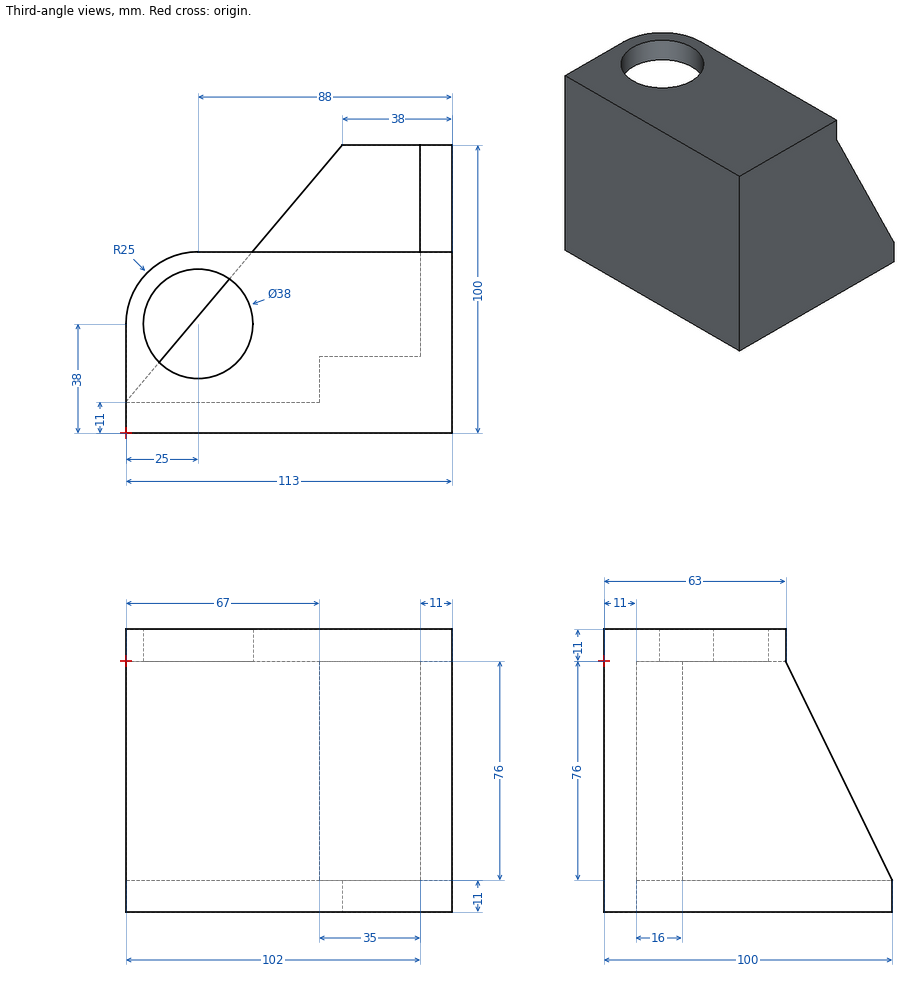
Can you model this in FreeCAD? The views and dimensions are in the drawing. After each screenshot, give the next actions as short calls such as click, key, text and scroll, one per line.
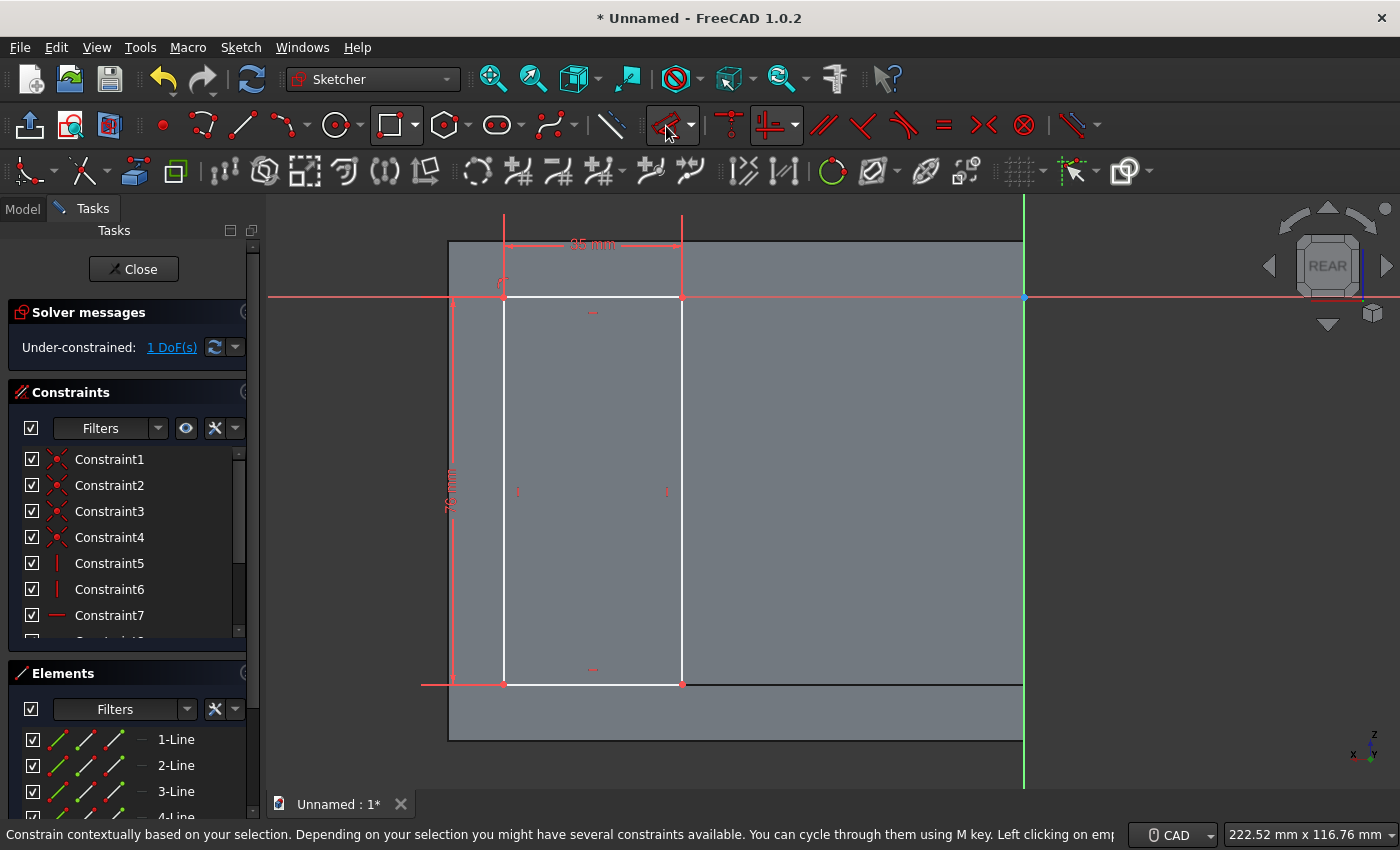
click(682, 685)
click(853, 719)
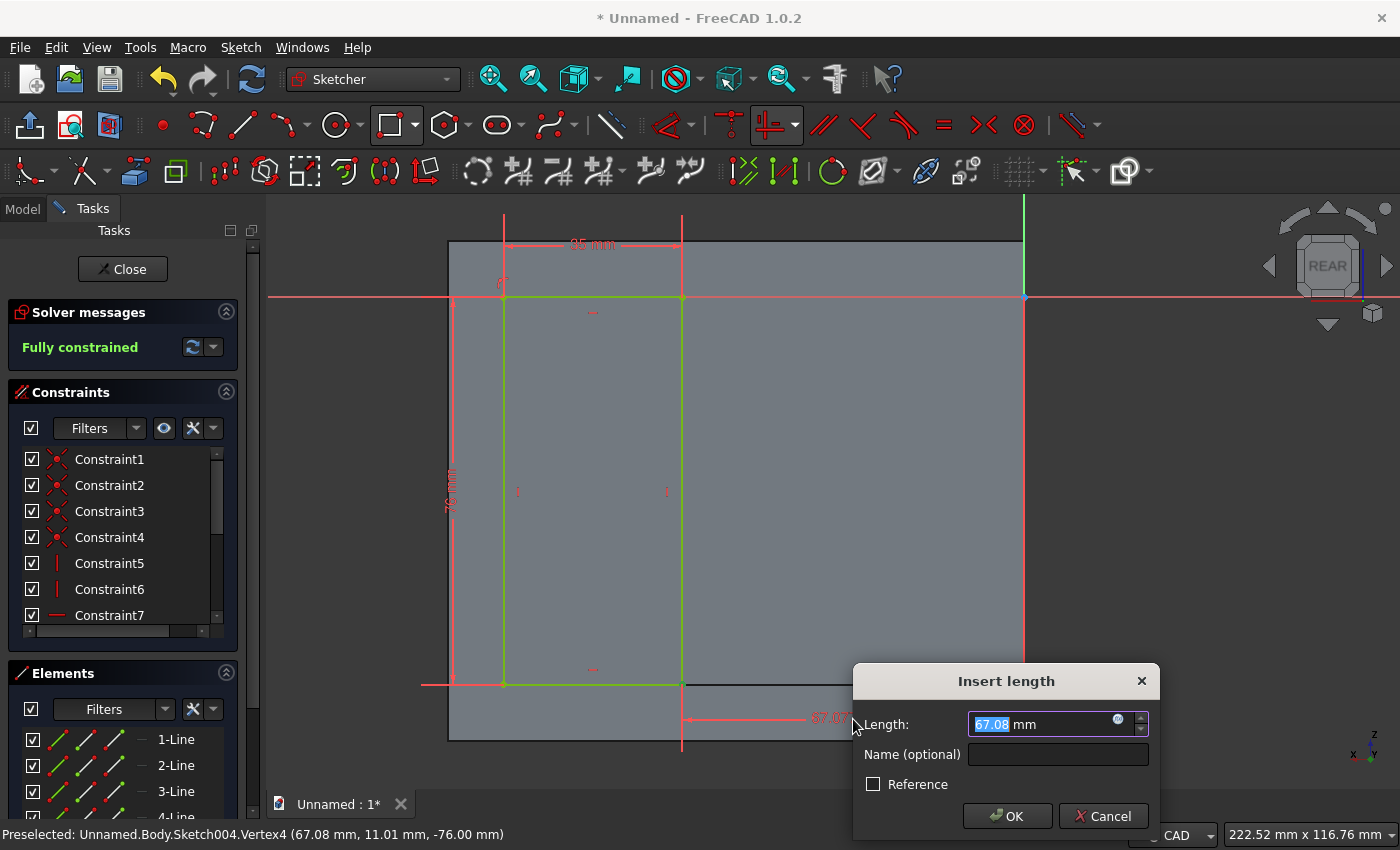
text(67)
key(Return)
key(Escape)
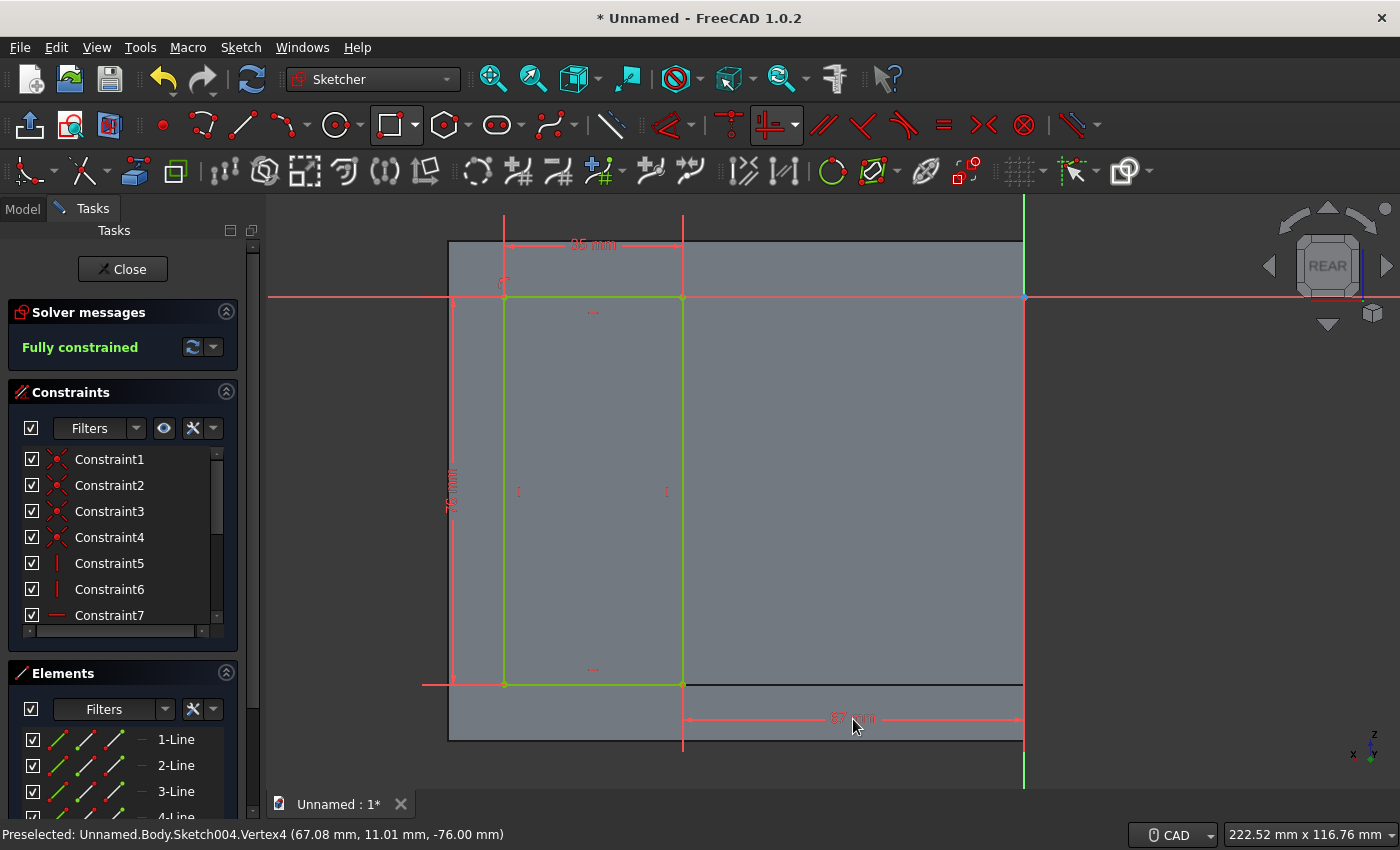
click(123, 269)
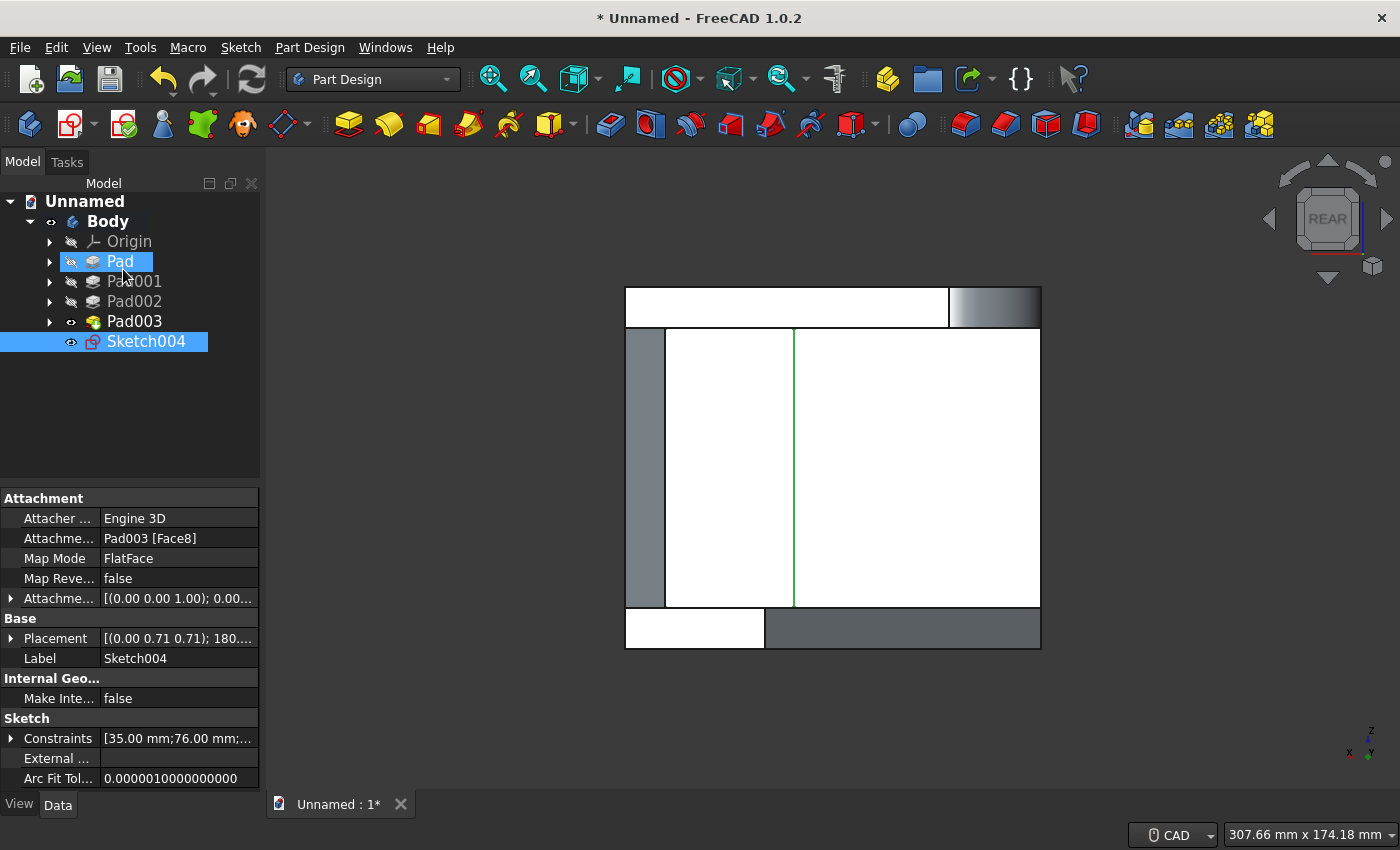
click(350, 124)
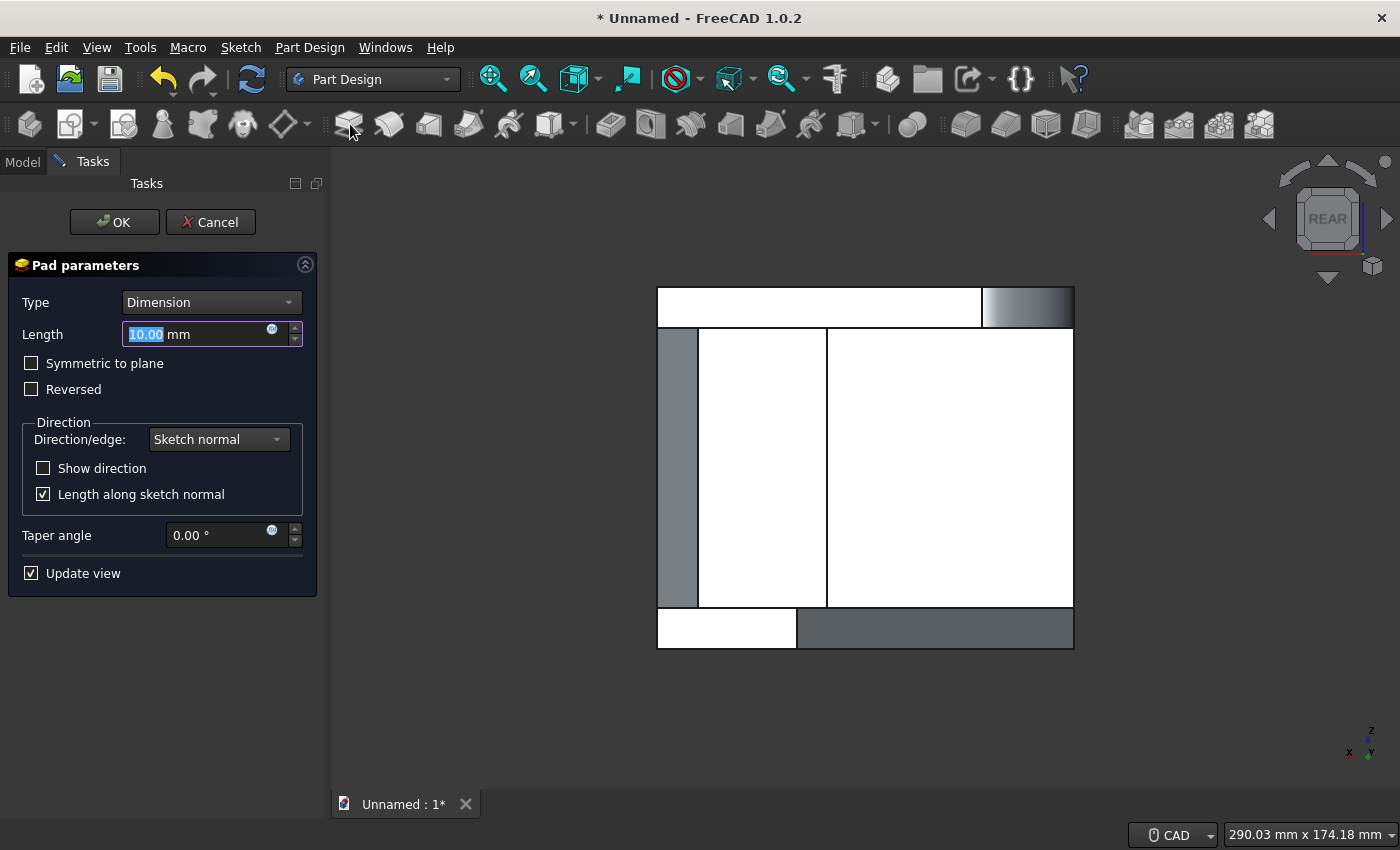
text(16)
key(Tab)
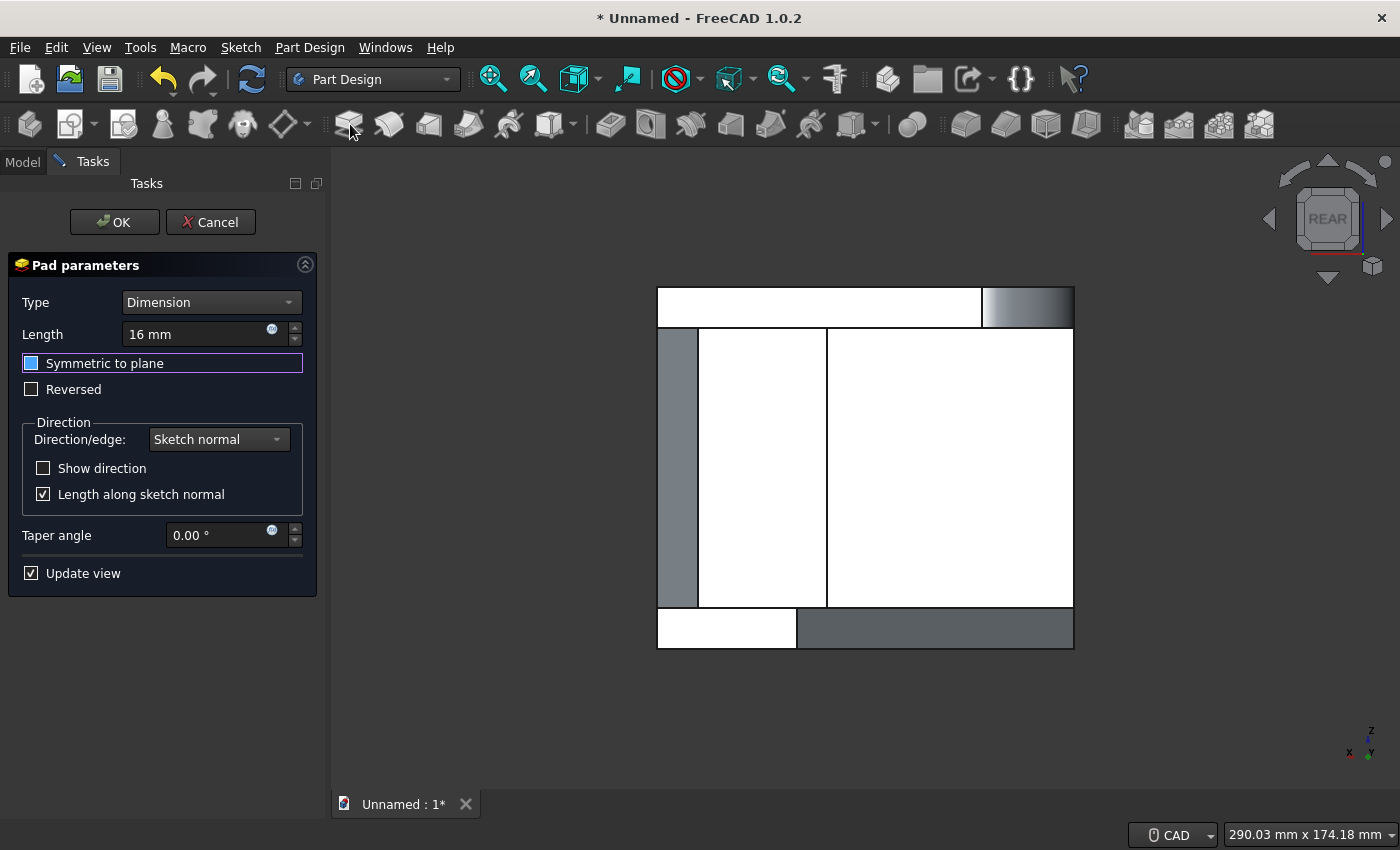
click(115, 222)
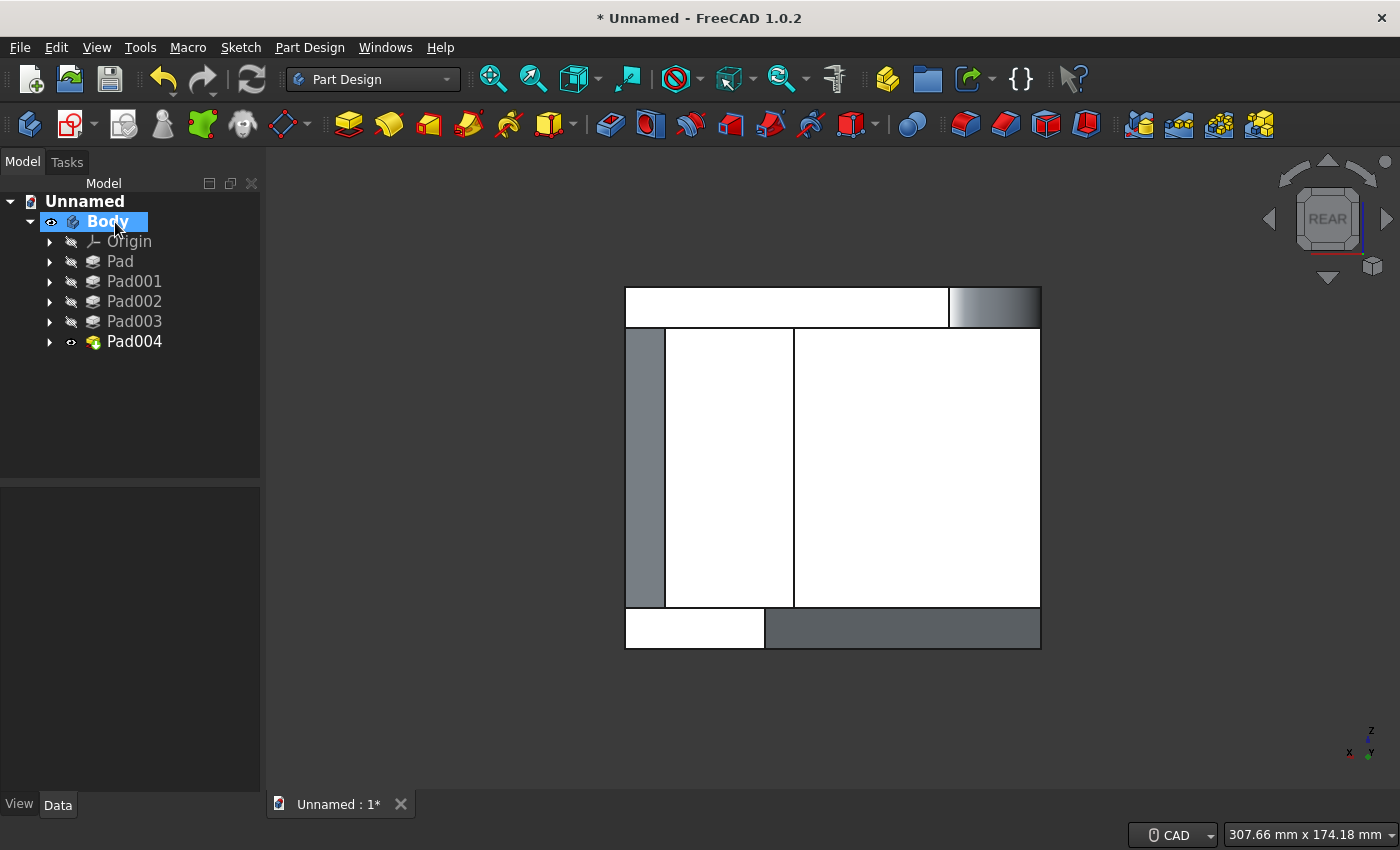
key(0)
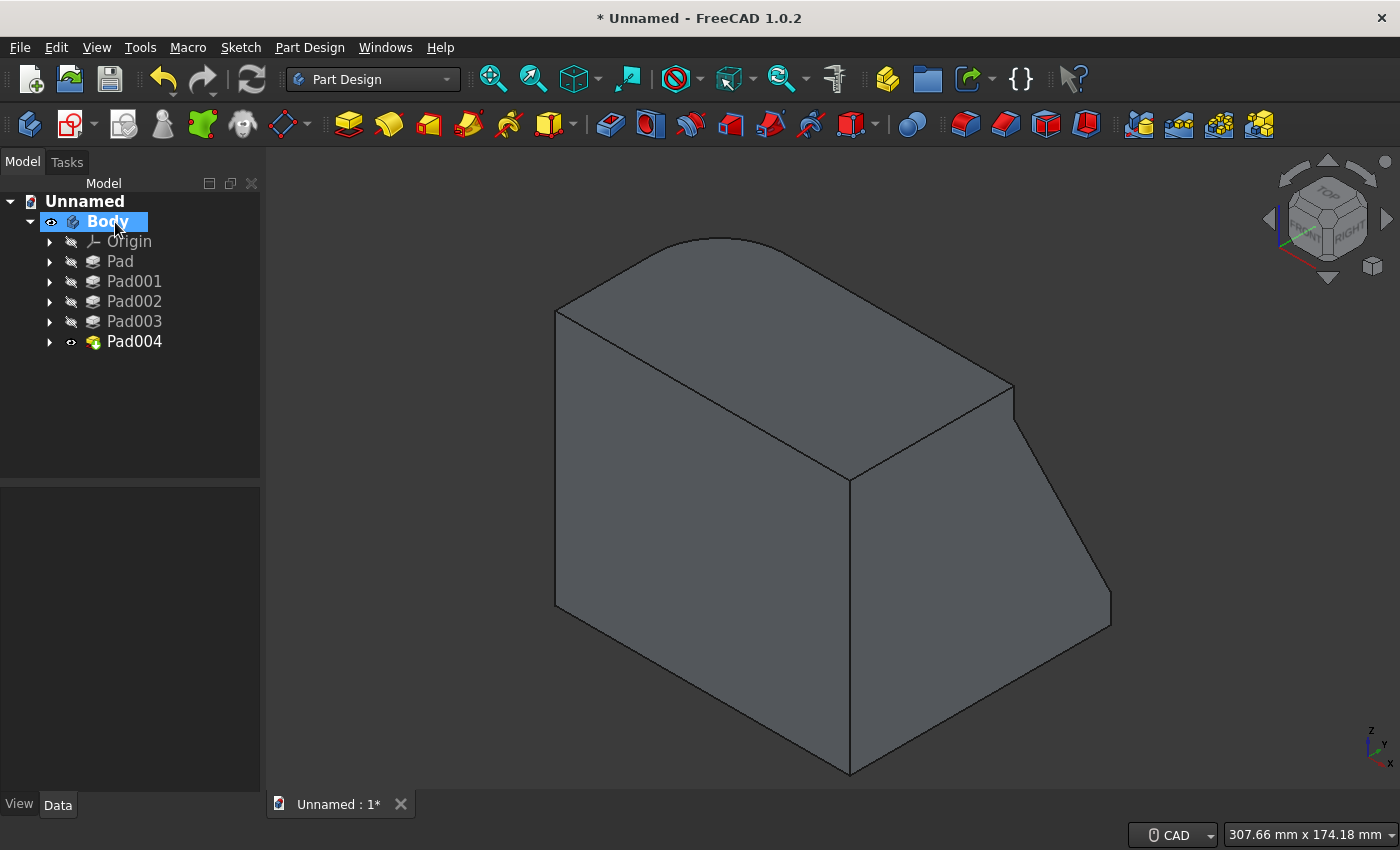
click(827, 372)